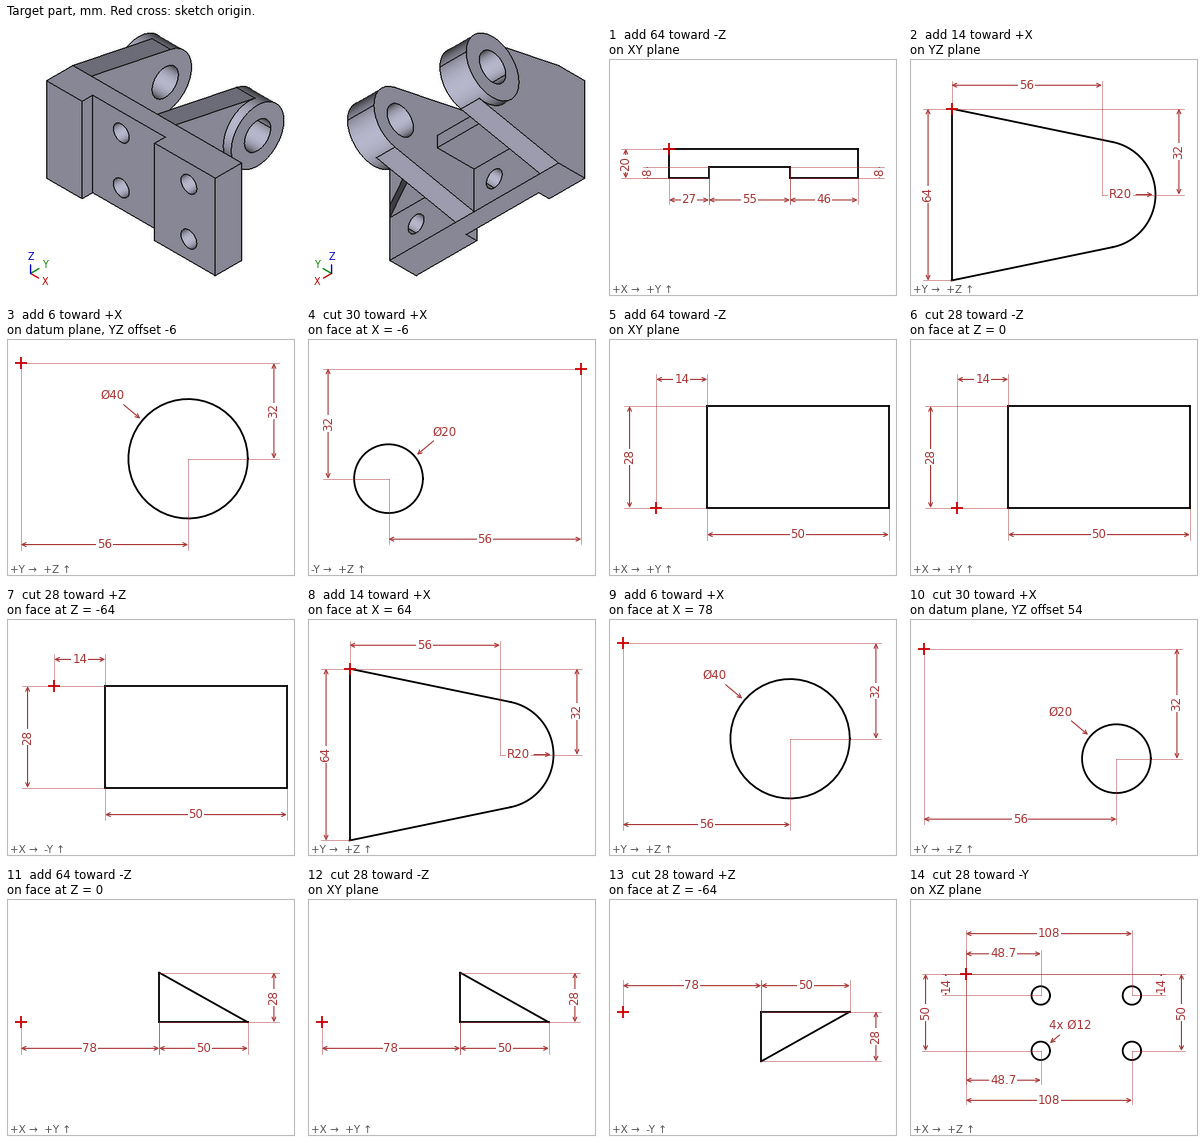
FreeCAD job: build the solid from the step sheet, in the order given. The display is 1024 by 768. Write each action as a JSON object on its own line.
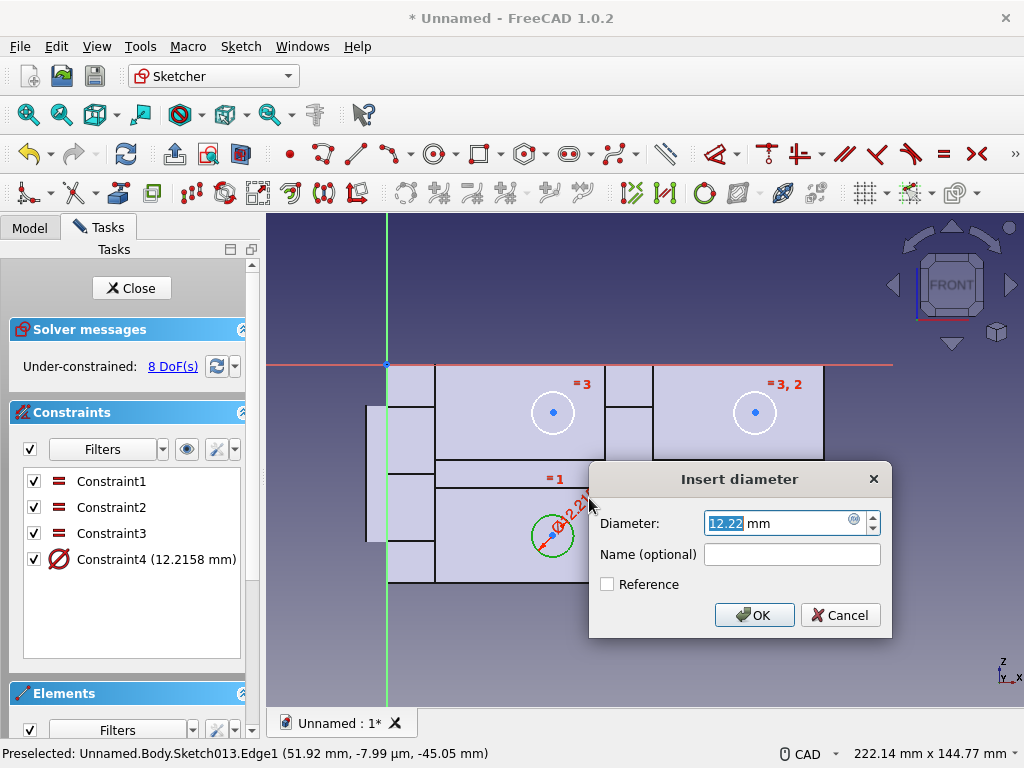
{"action": "type", "text": "12"}
{"action": "key", "text": "Return"}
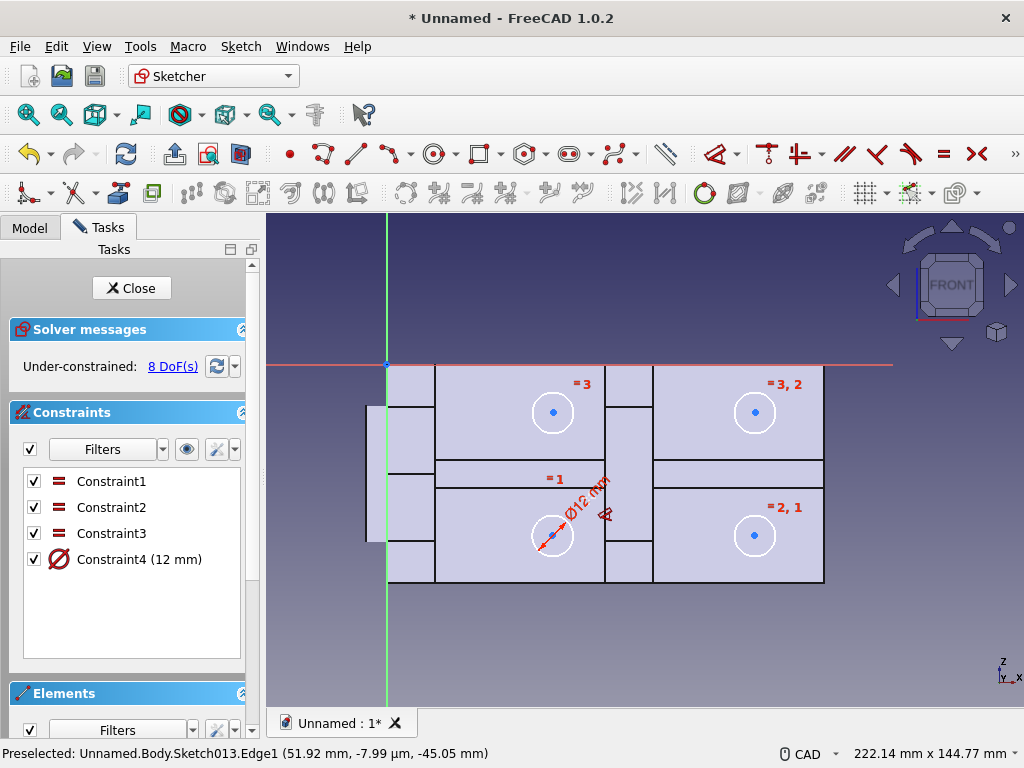
{"action": "left_click", "coordinate": [553, 536]}
{"action": "left_click", "coordinate": [353, 450]}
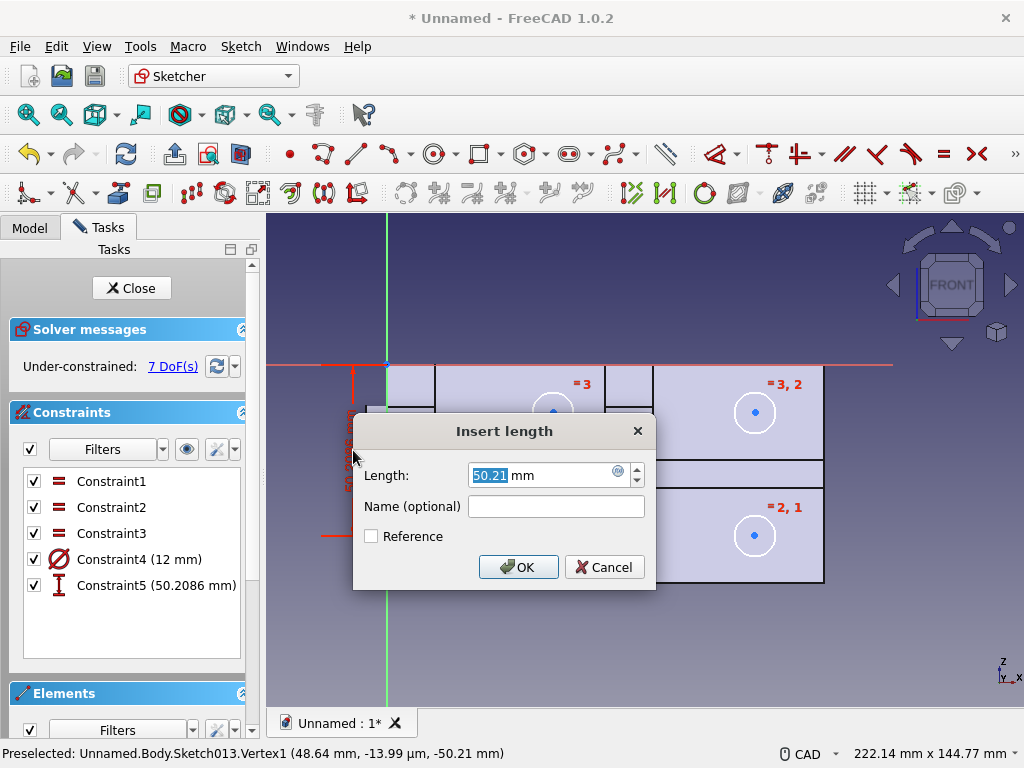
{"action": "type", "text": "50"}
{"action": "key", "text": "Return"}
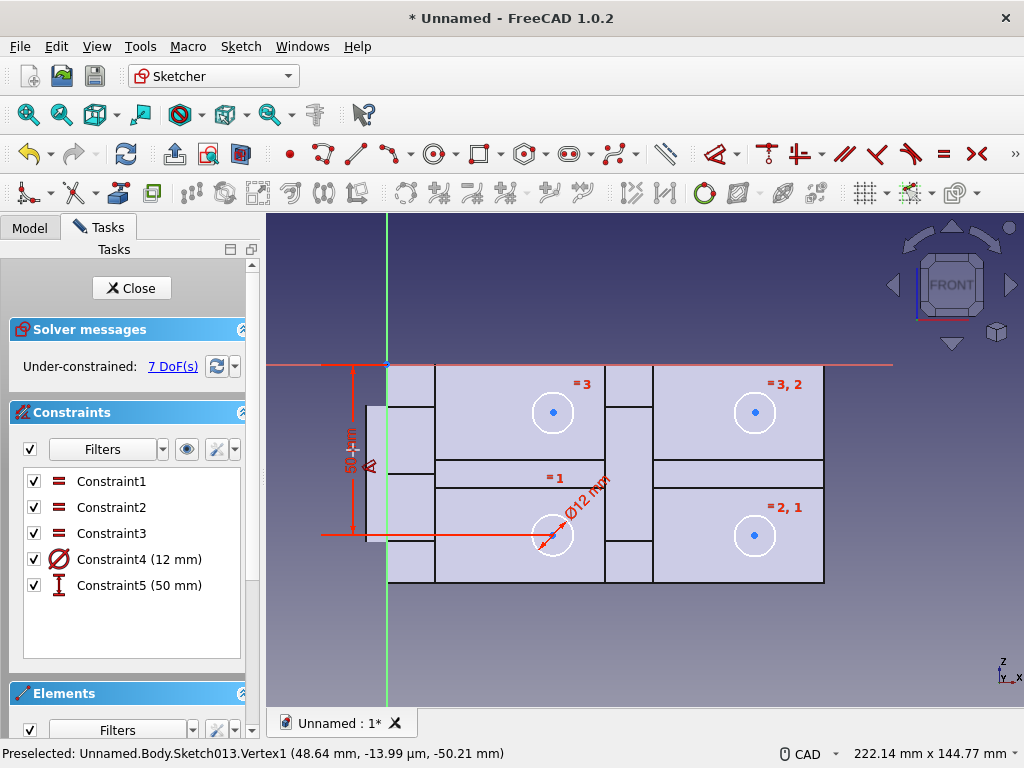
{"action": "left_click", "coordinate": [755, 536]}
{"action": "left_click", "coordinate": [353, 411]}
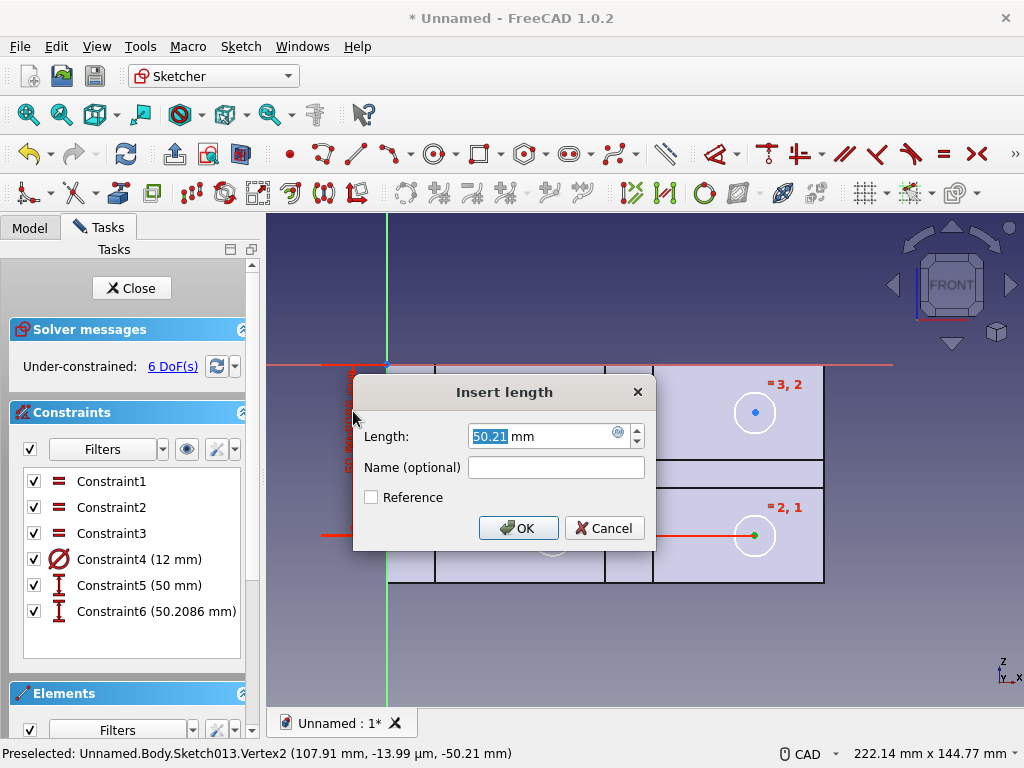
{"action": "type", "text": "50"}
{"action": "key", "text": "Return"}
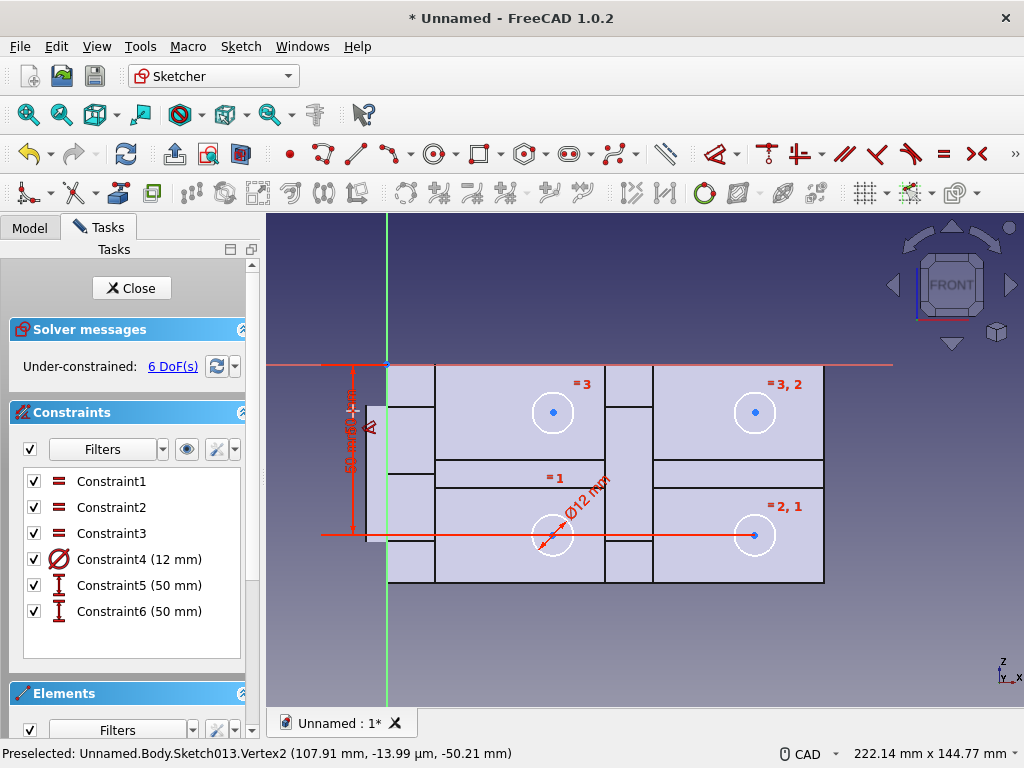
{"action": "left_click", "coordinate": [755, 413]}
{"action": "left_click", "coordinate": [353, 389]}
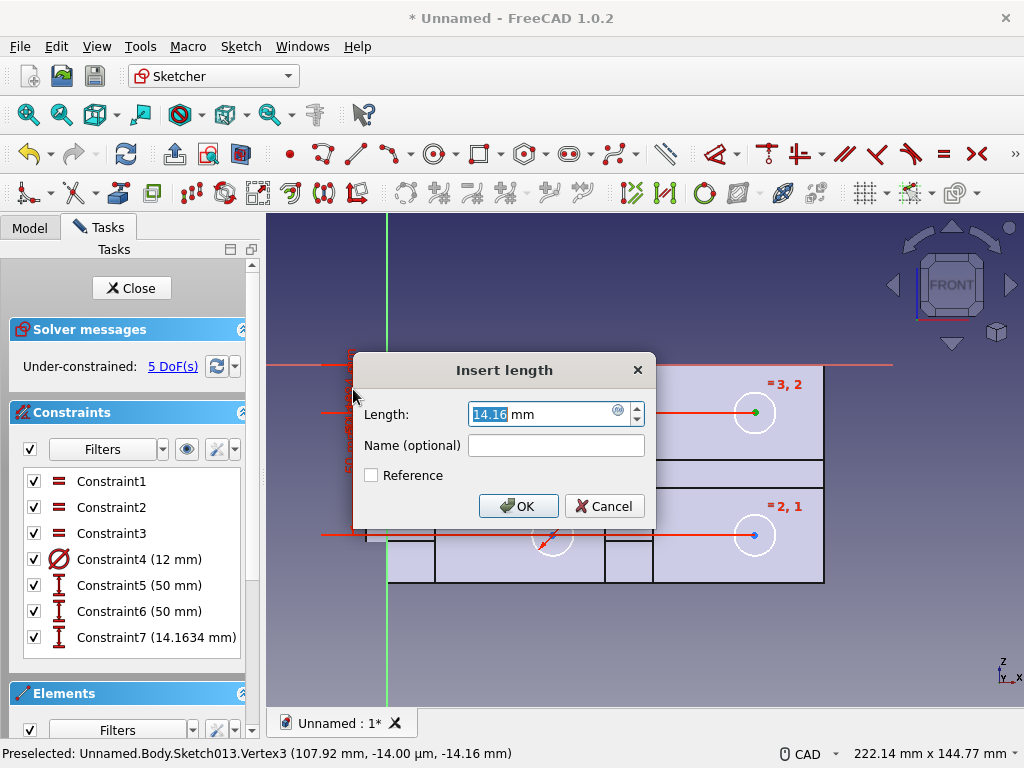
{"action": "type", "text": "14"}
{"action": "key", "text": "Return"}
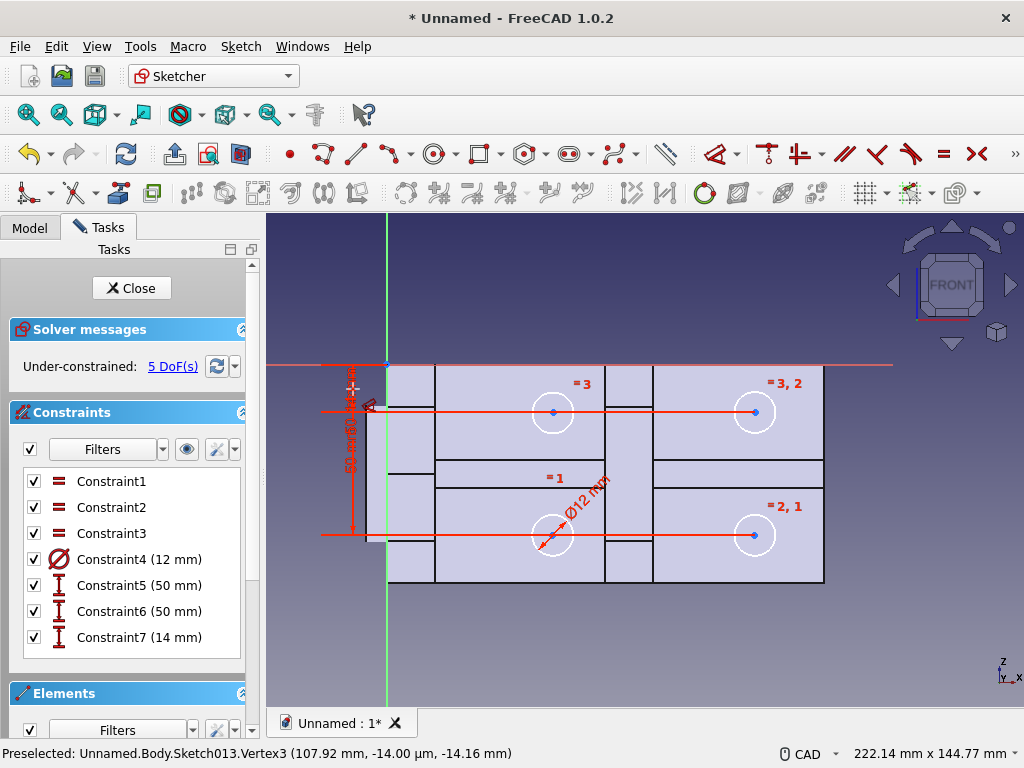
{"action": "left_click", "coordinate": [553, 413]}
{"action": "left_click", "coordinate": [587, 389]}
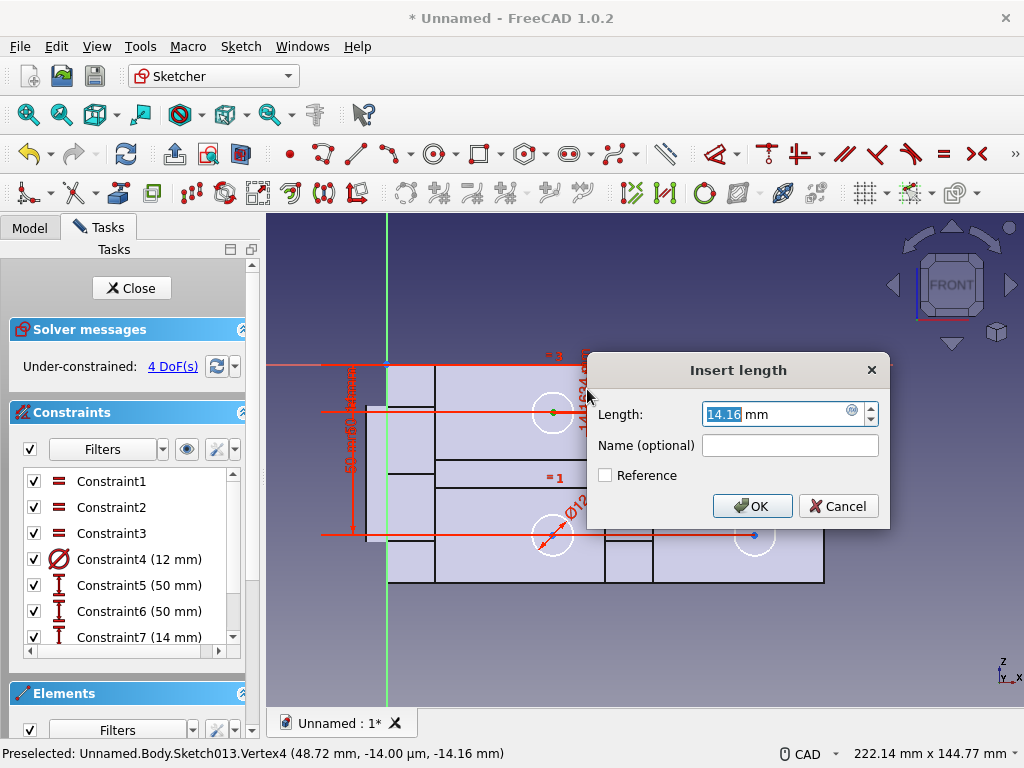
{"action": "type", "text": "14"}
{"action": "key", "text": "Return"}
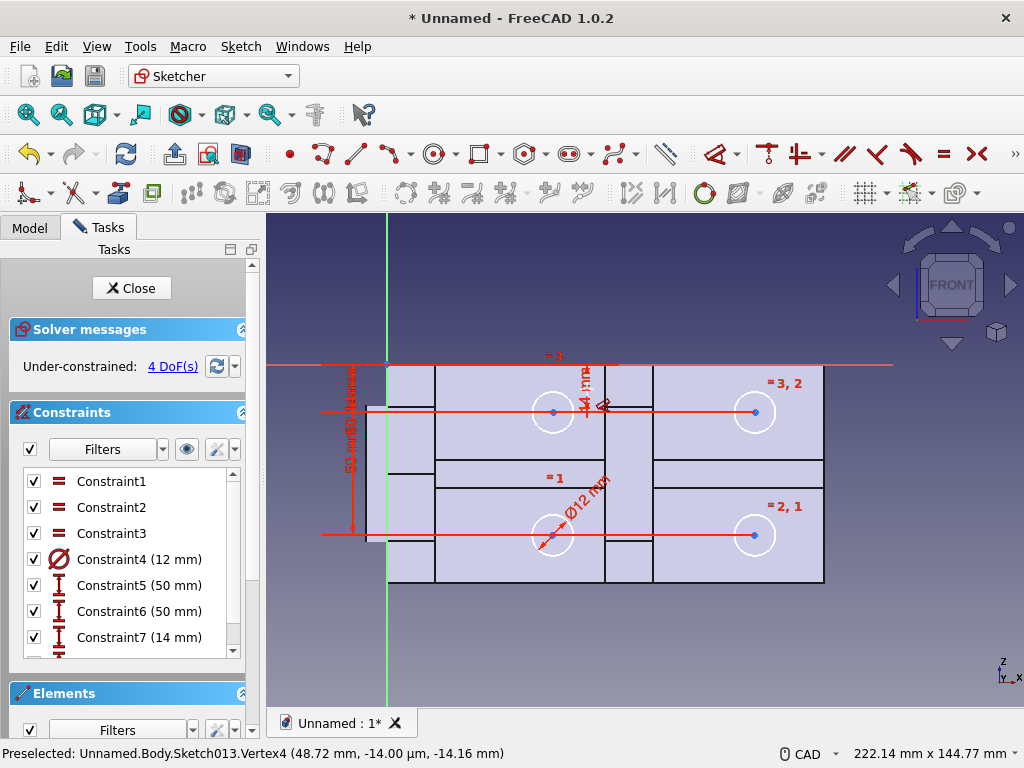
{"action": "left_click", "coordinate": [755, 535]}
{"action": "left_click", "coordinate": [571, 331]}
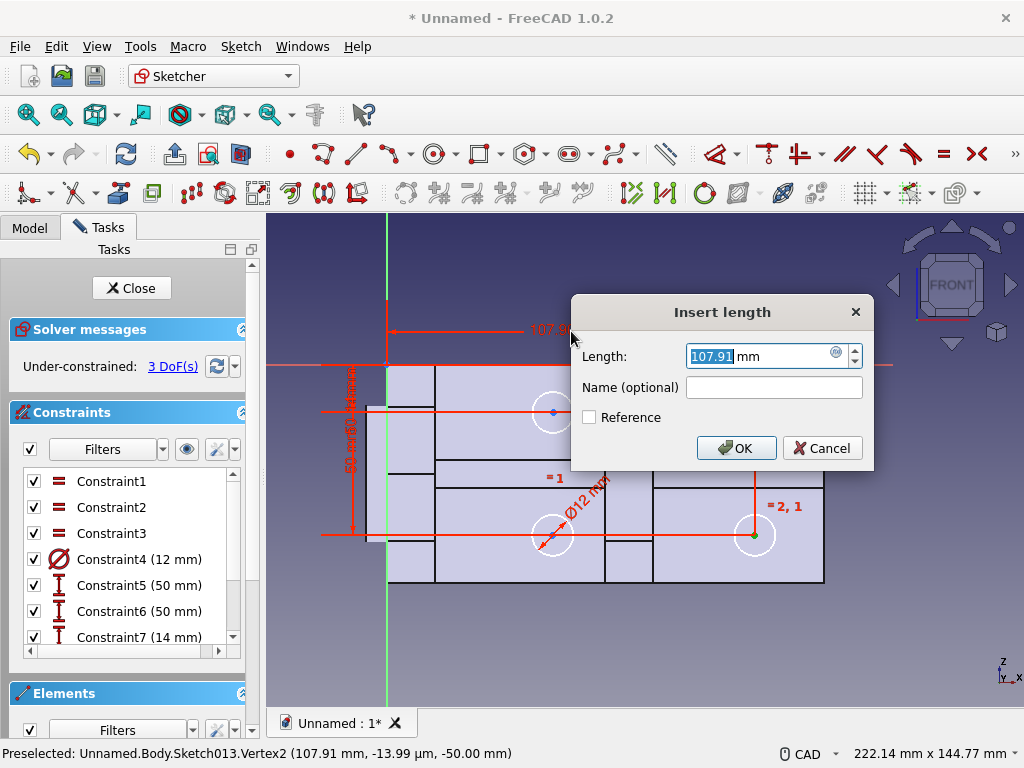
{"action": "type", "text": "108"}
{"action": "key", "text": "Return"}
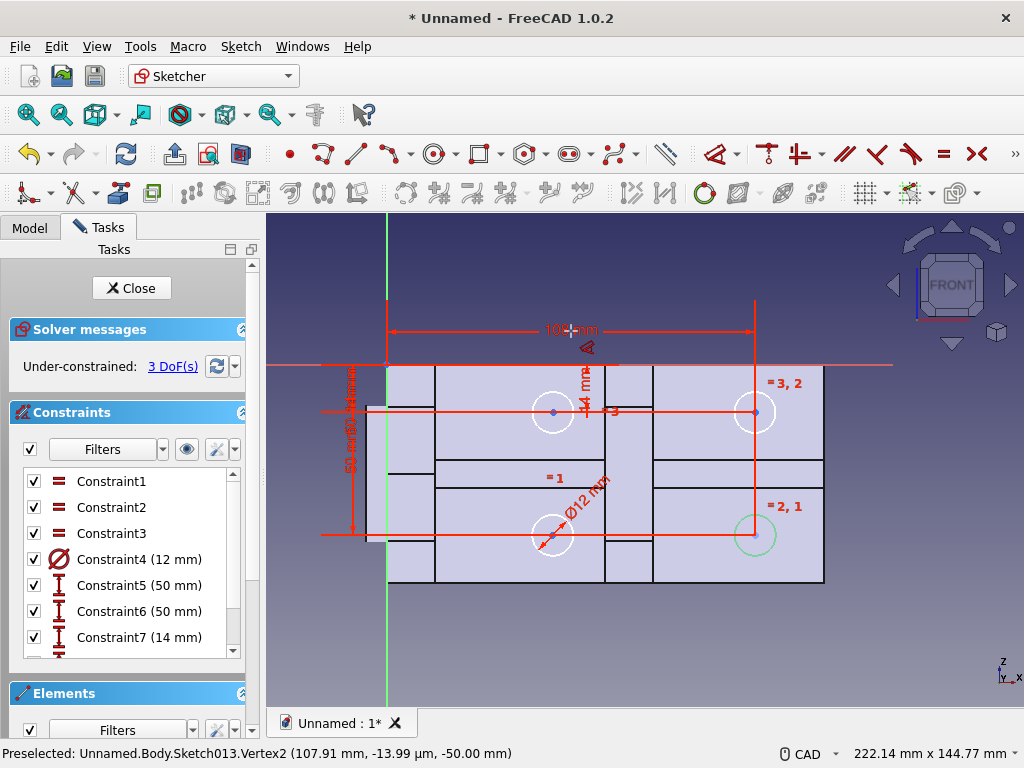
{"action": "left_click", "coordinate": [755, 412]}
{"action": "left_click", "coordinate": [486, 331]}